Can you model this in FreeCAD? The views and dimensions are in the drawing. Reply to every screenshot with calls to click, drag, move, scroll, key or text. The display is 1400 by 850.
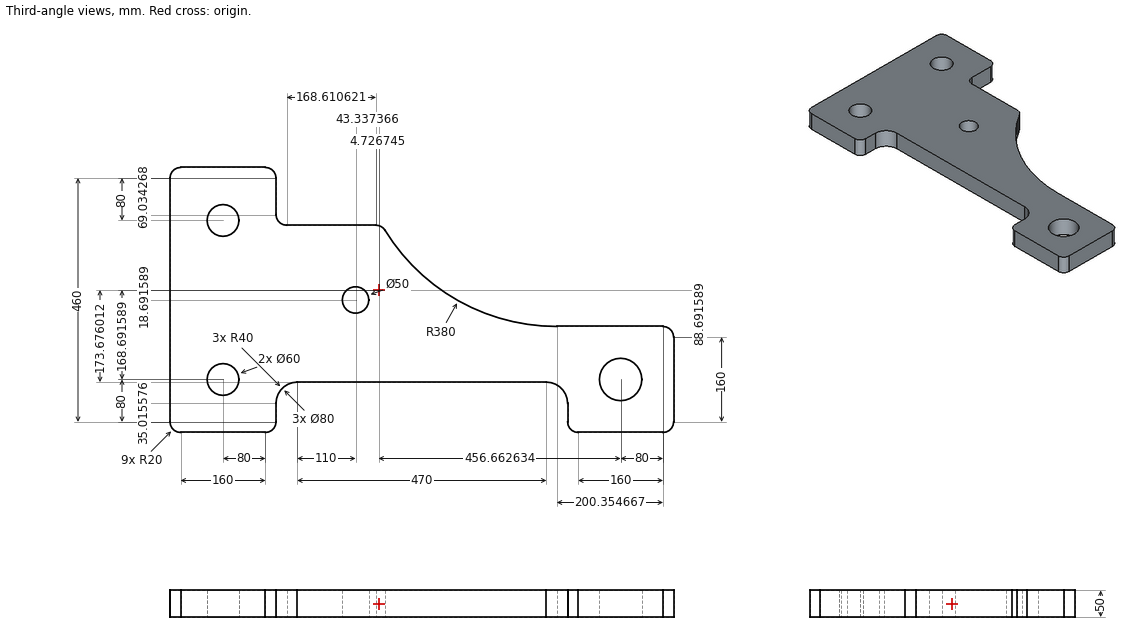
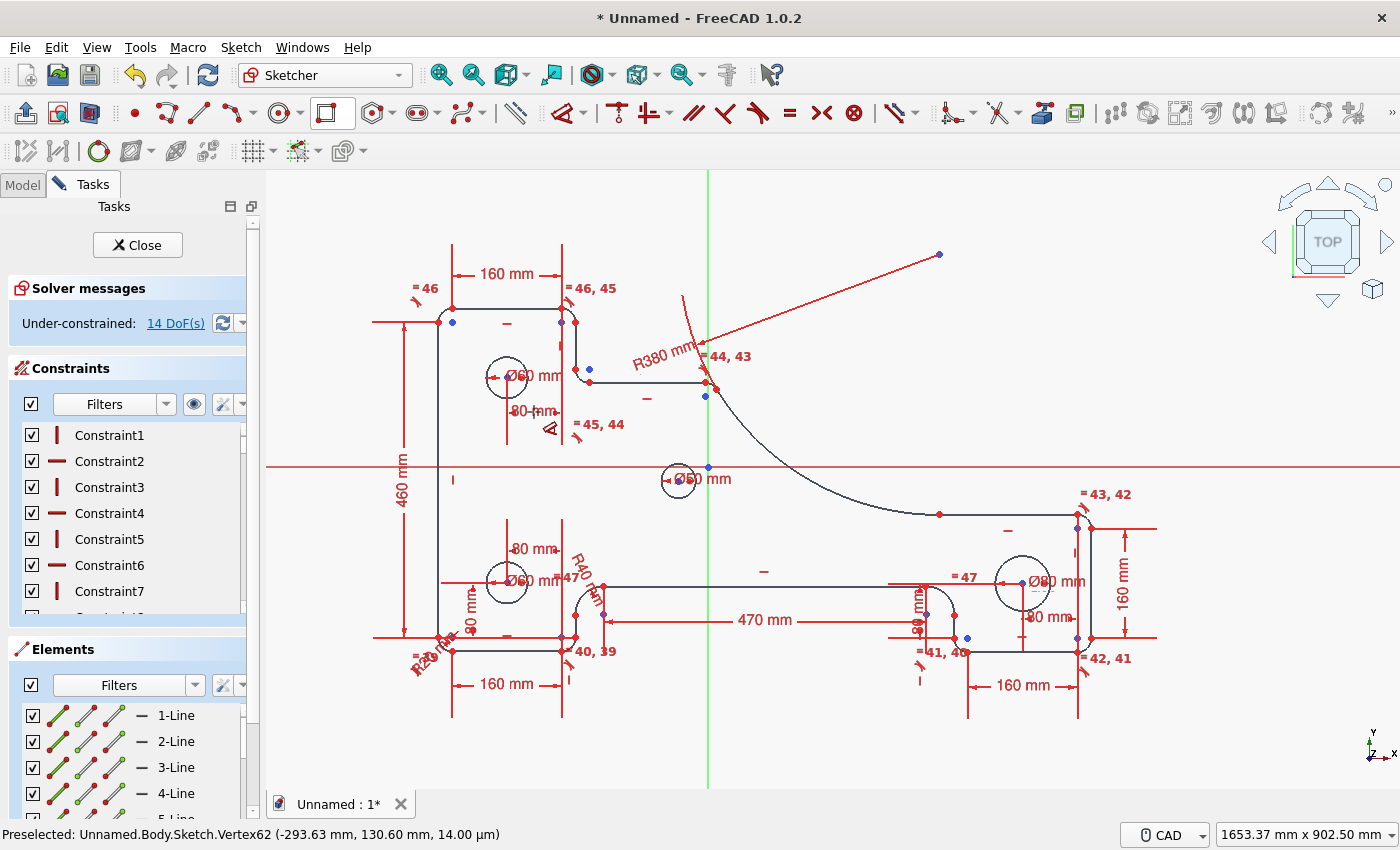
click(576, 322)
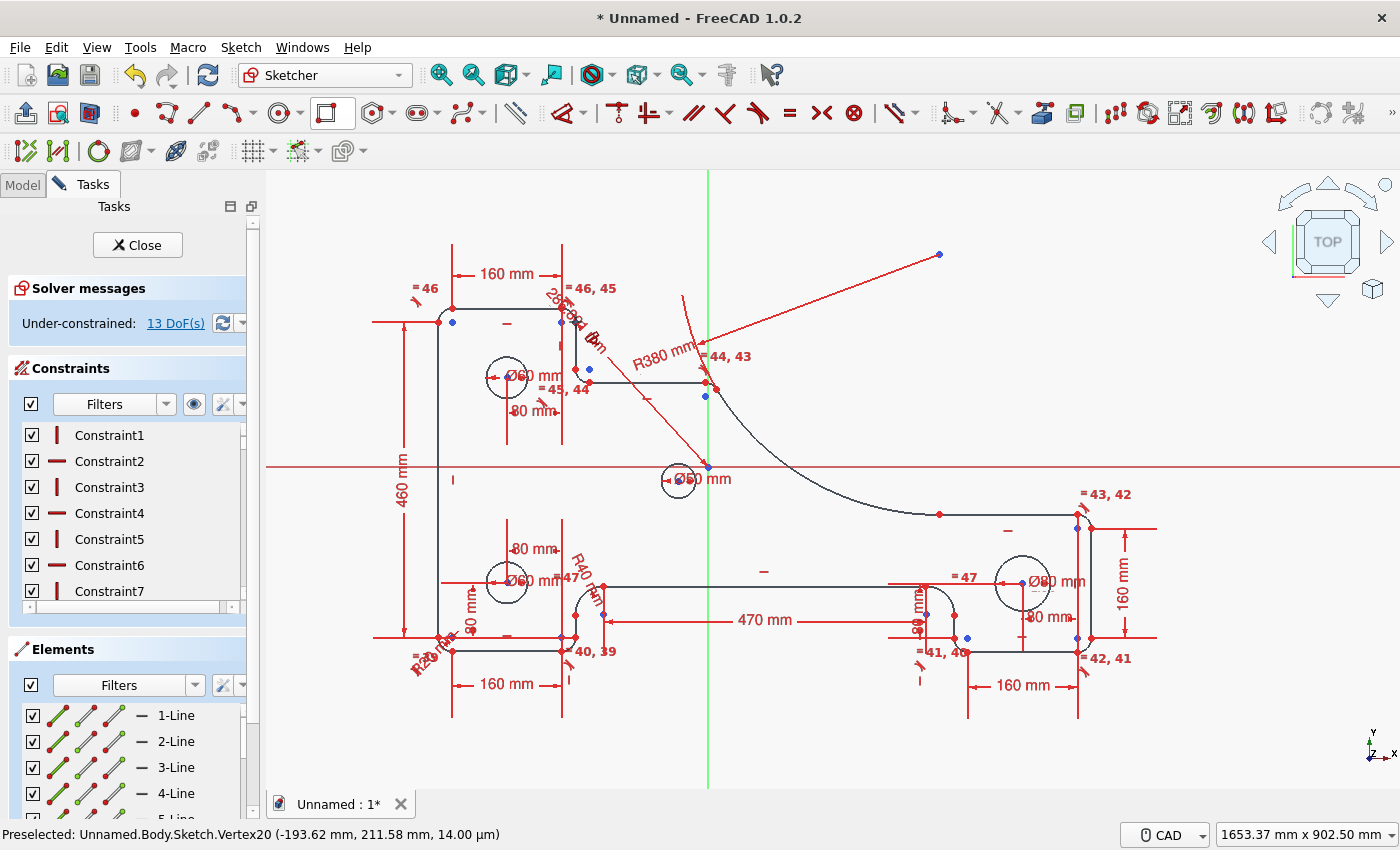
click(507, 378)
click(473, 350)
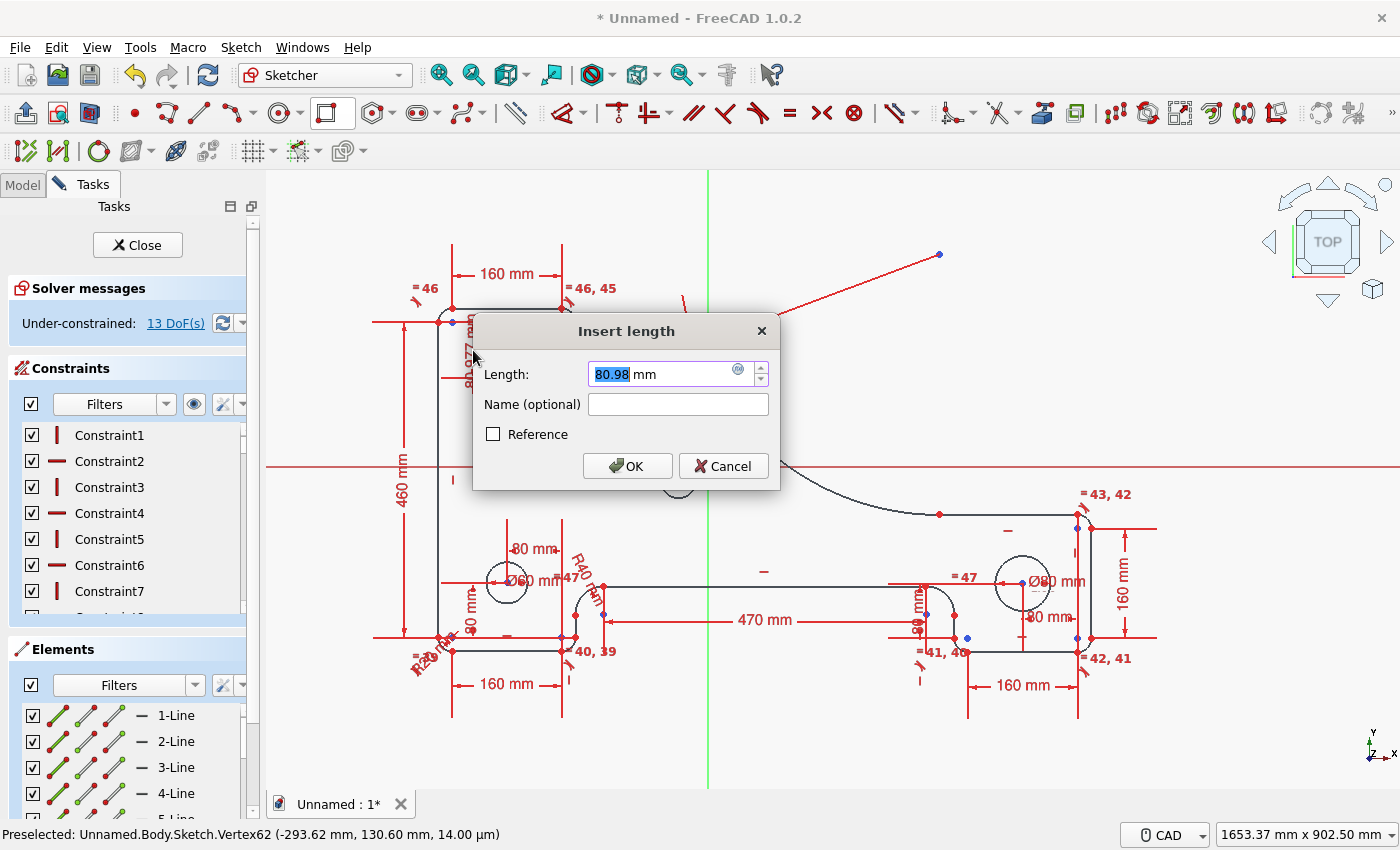
text(80)
key(Return)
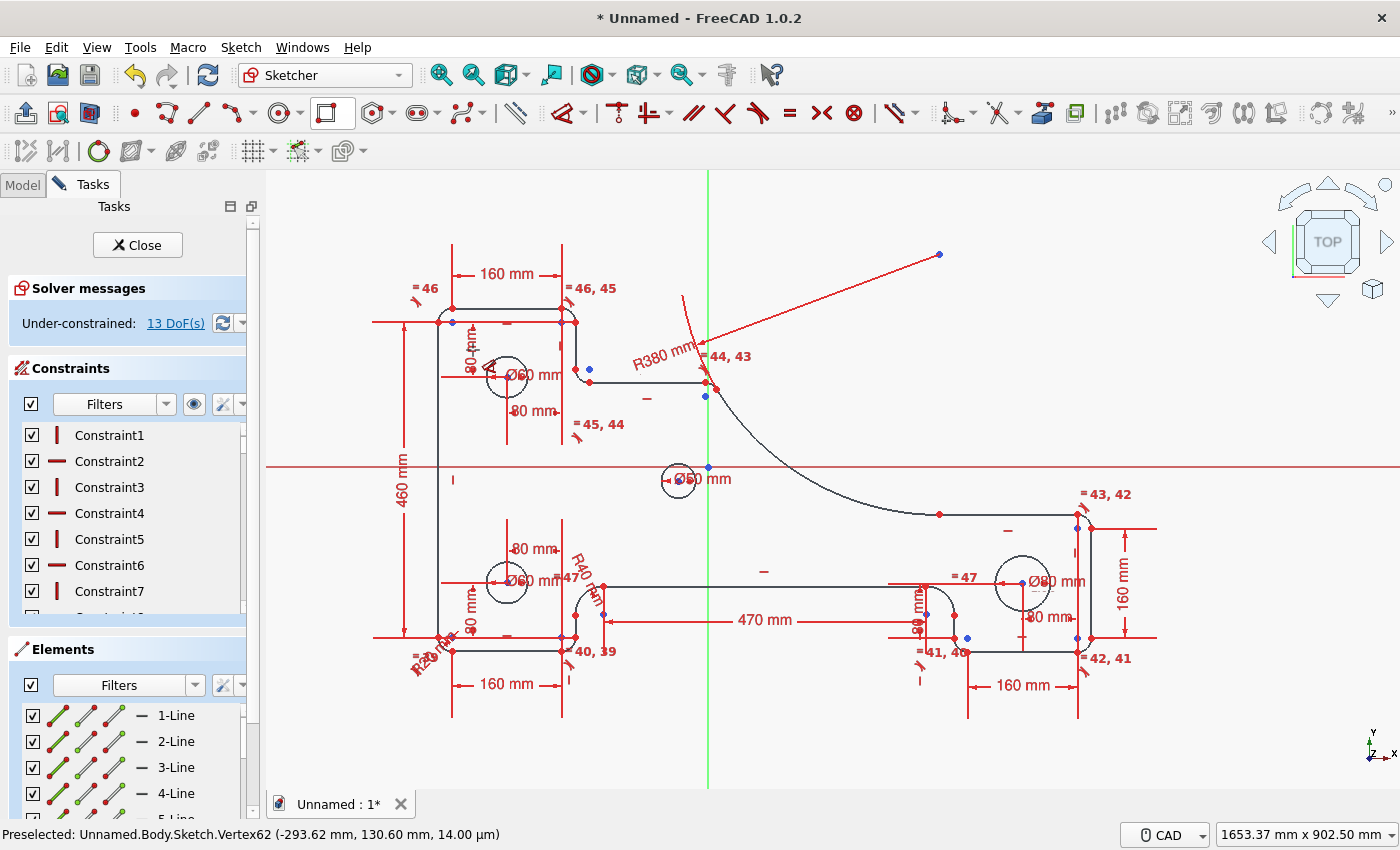
click(604, 587)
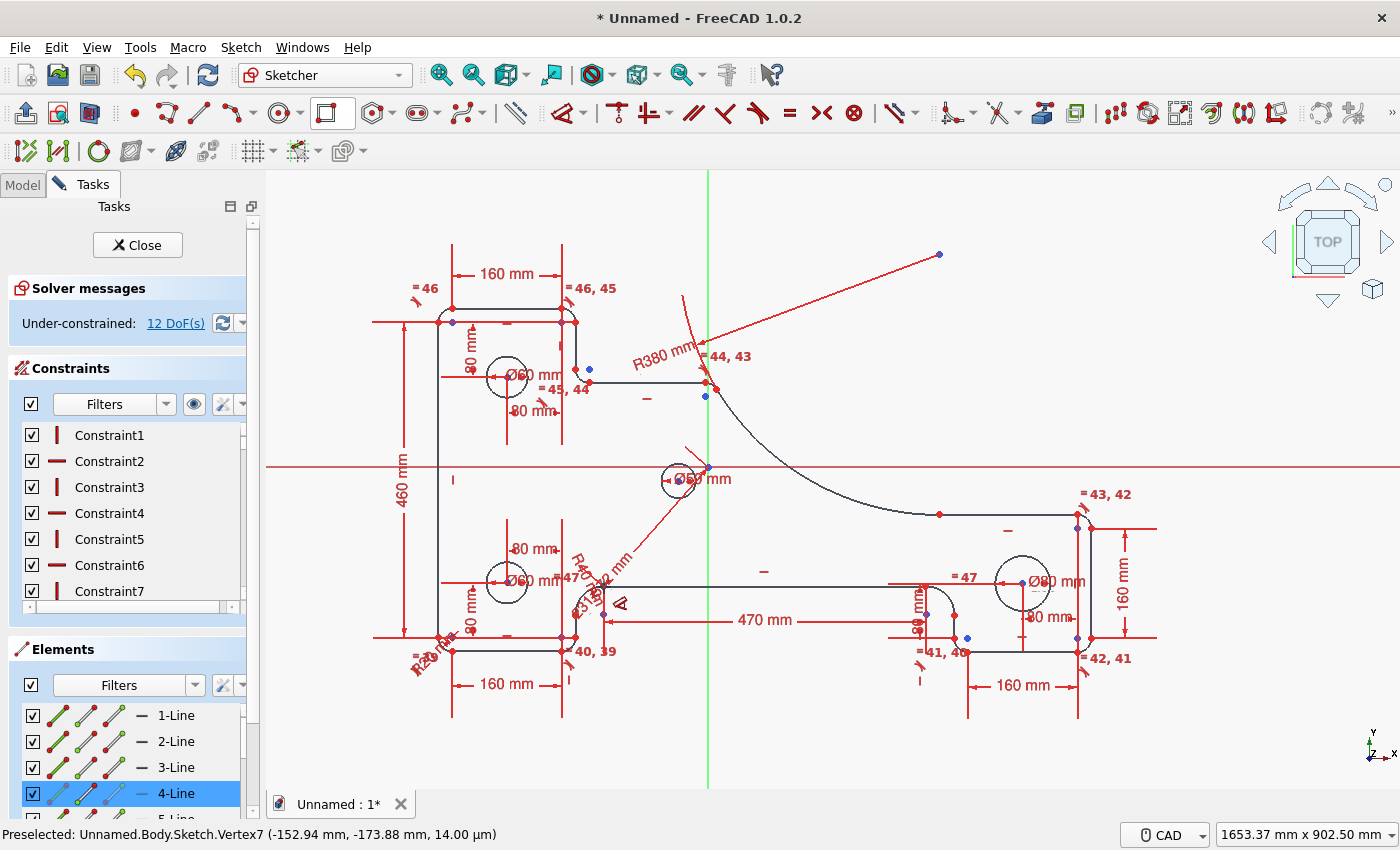
click(679, 481)
click(641, 621)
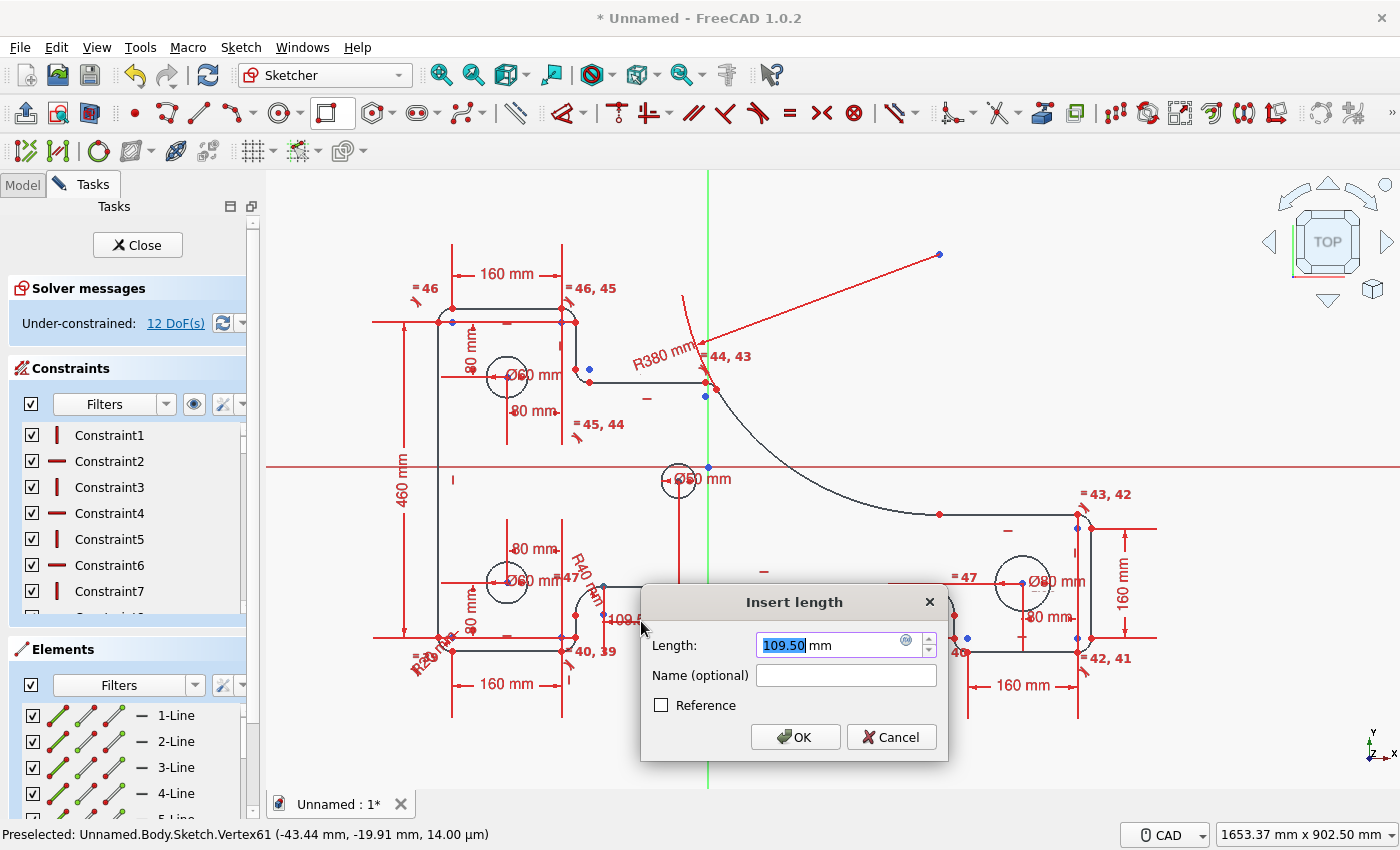
text(110)
key(Return)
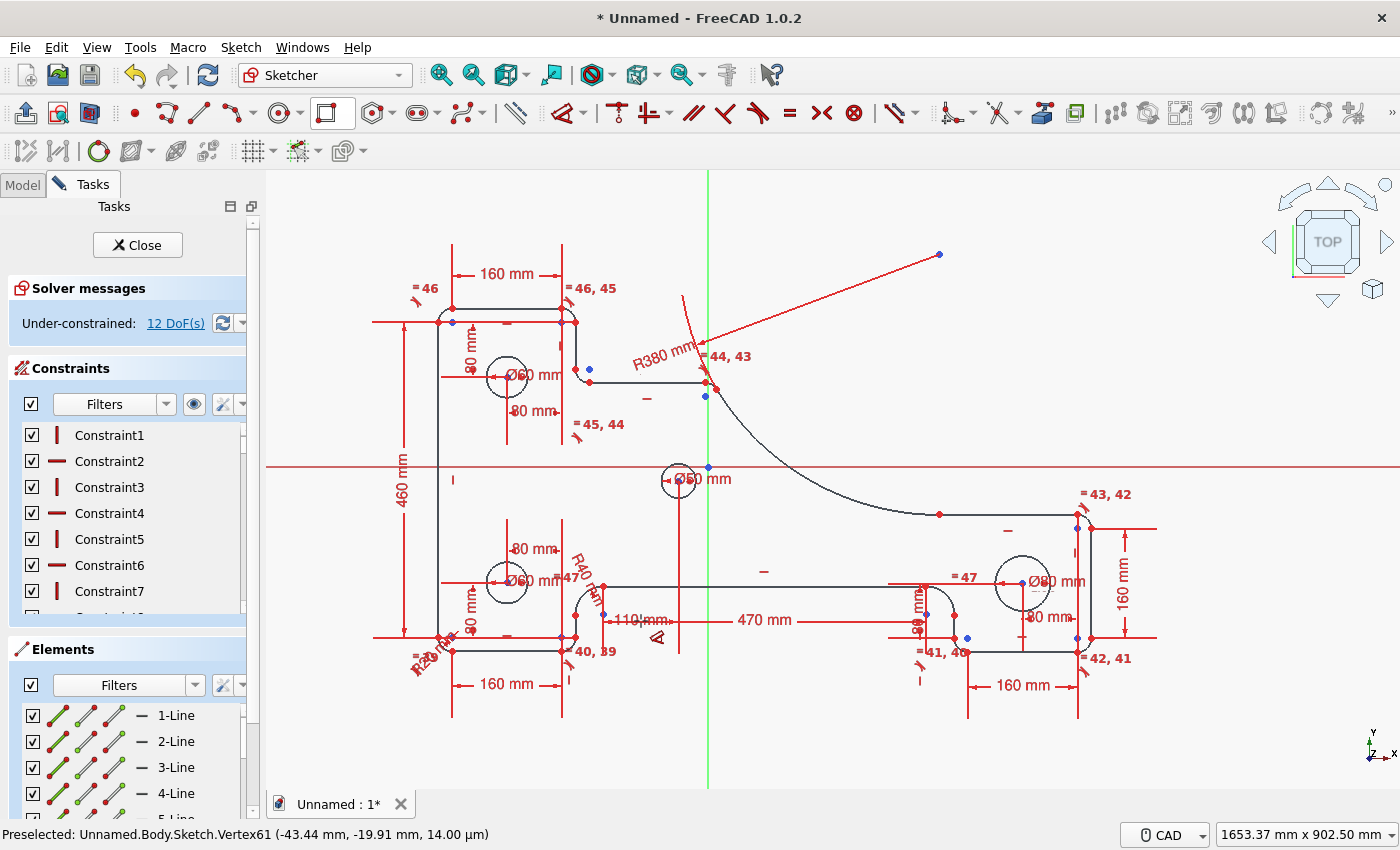
scroll(576, 627, up, 3)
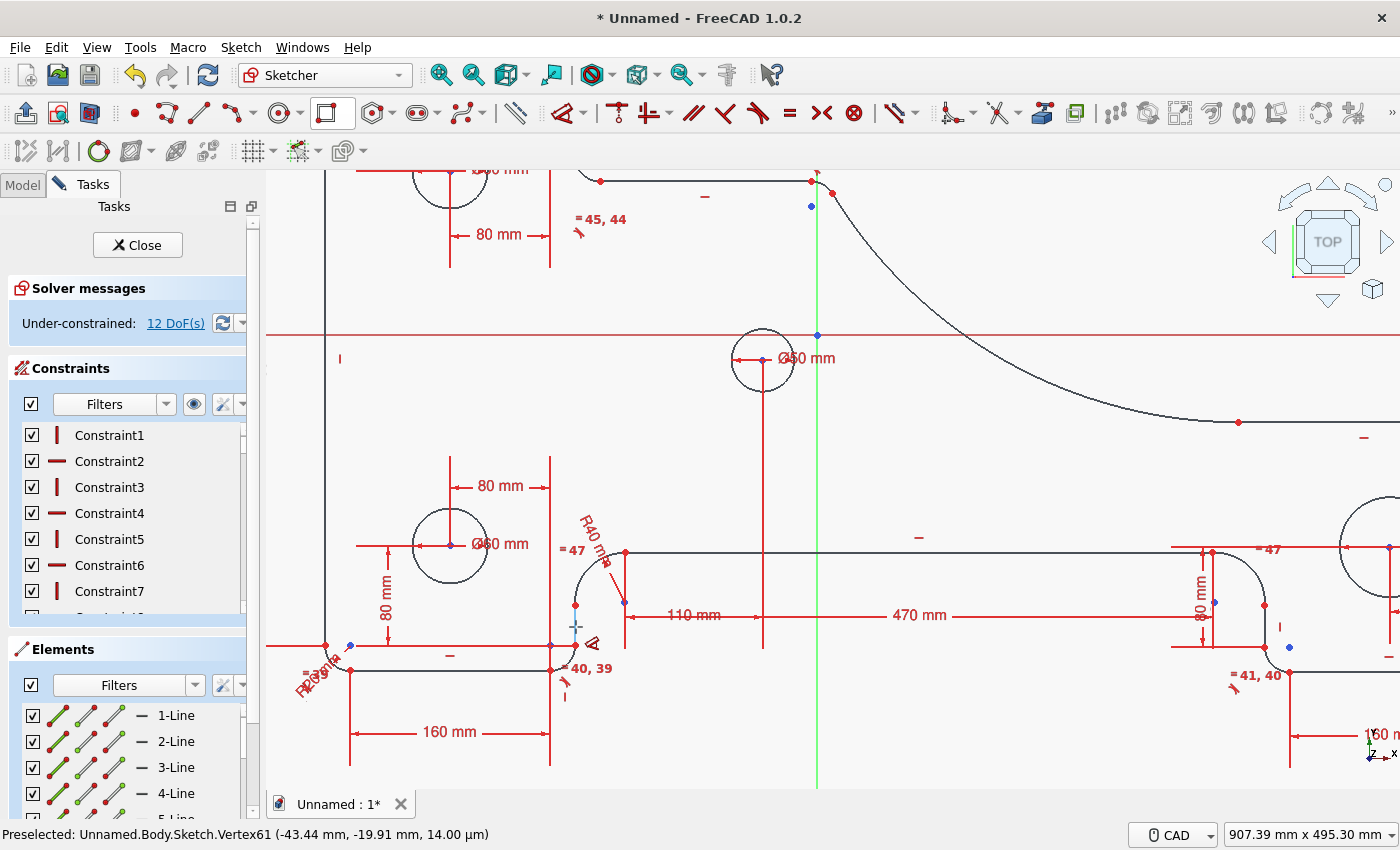
click(575, 626)
click(541, 626)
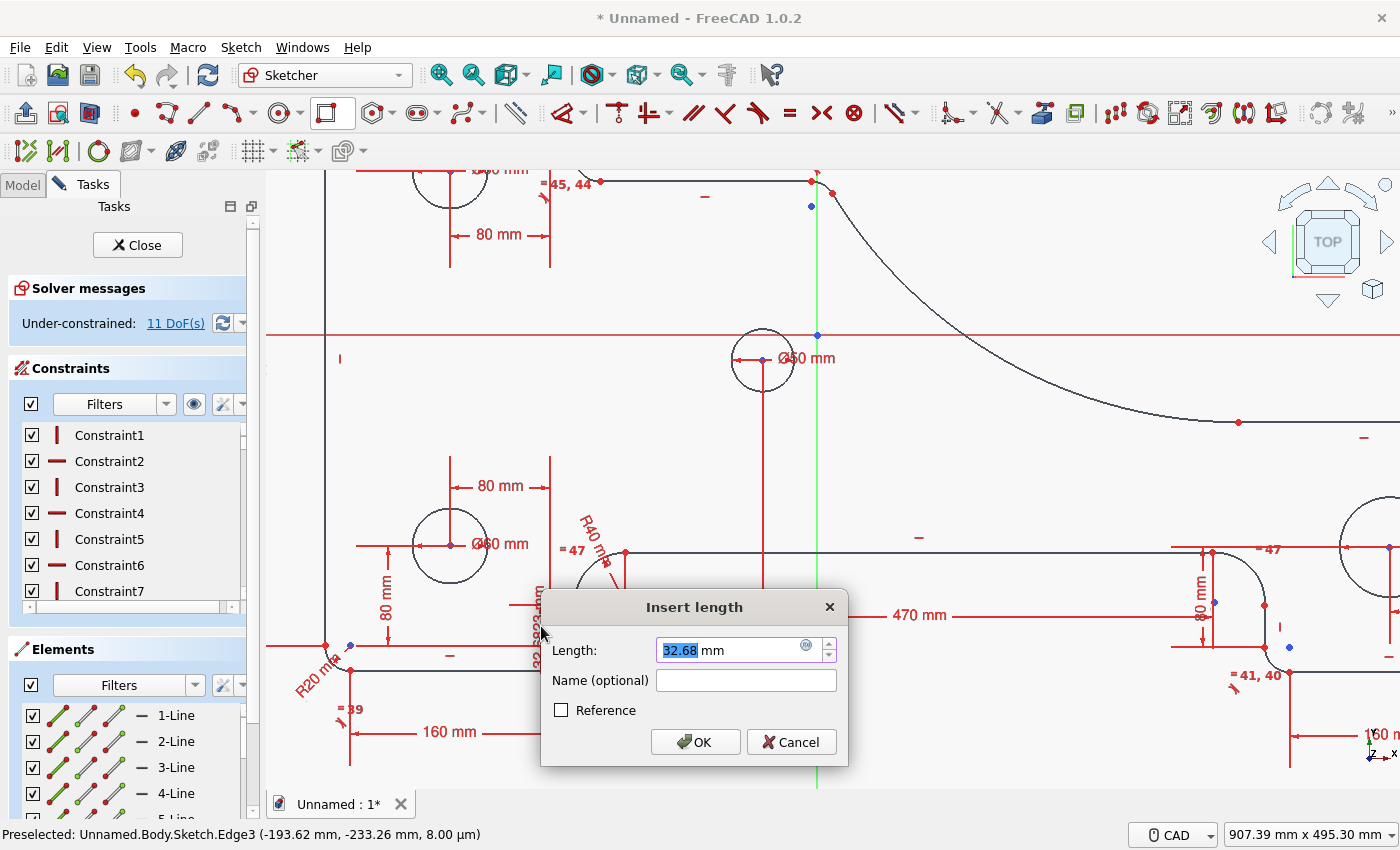
text(35.015576)
key(Return)